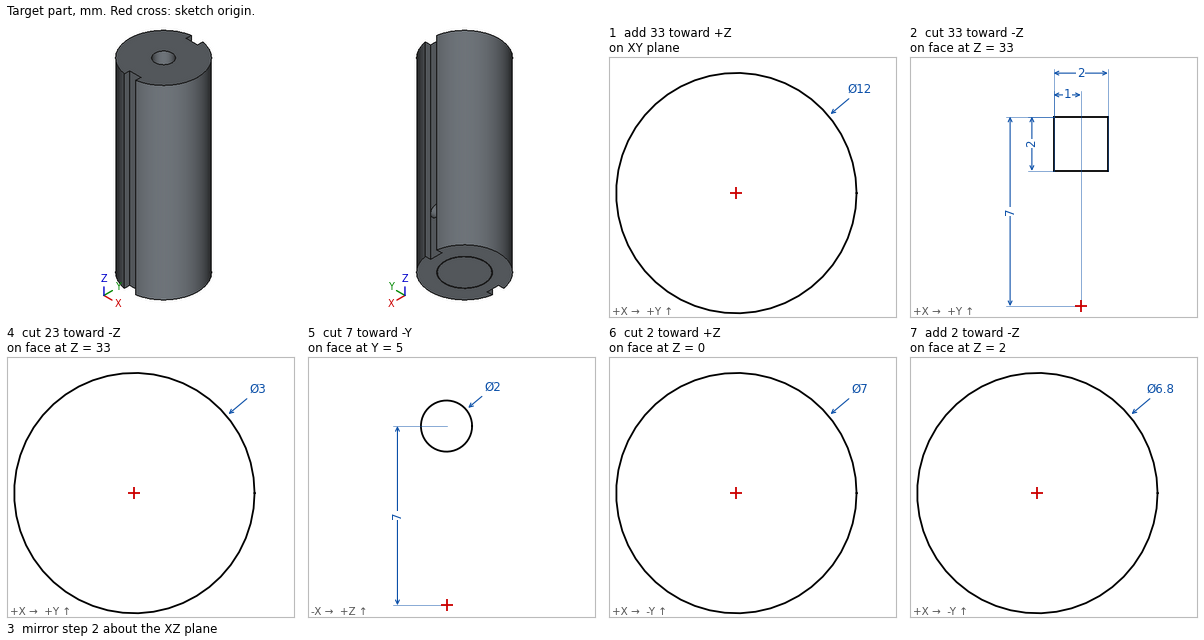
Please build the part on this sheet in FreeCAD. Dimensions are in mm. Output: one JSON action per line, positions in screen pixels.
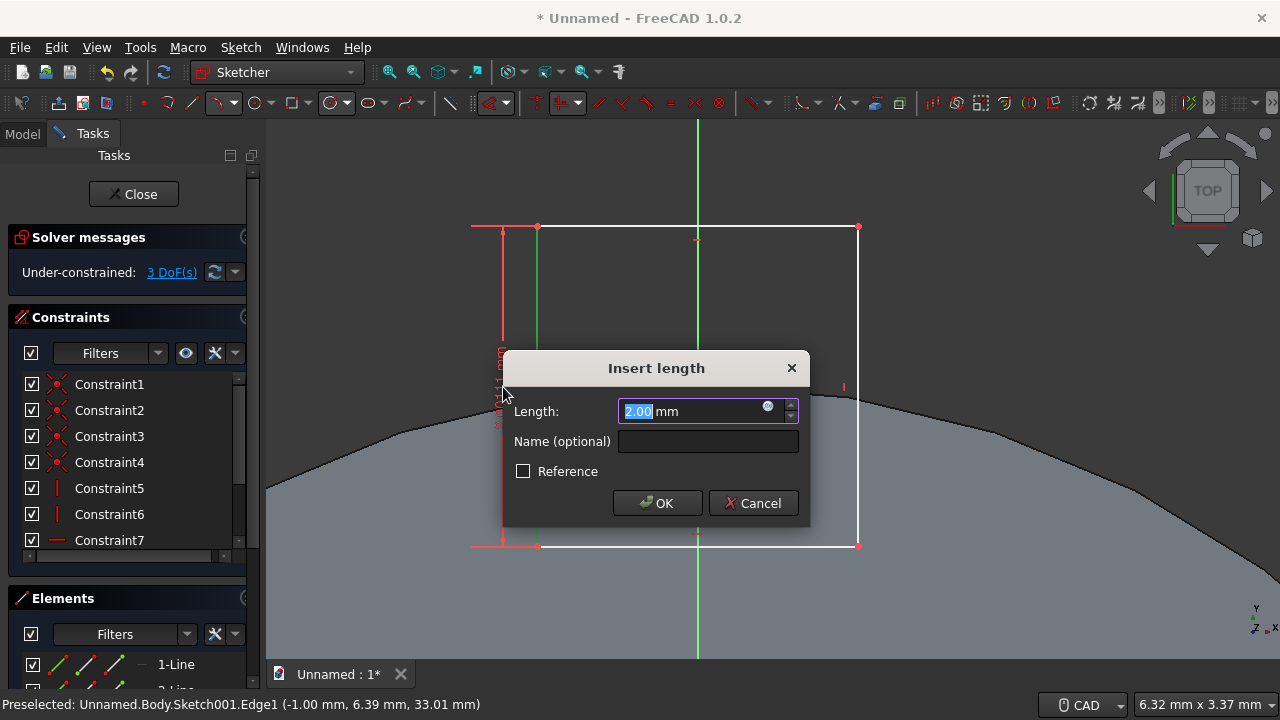
{"action": "type", "text": "2"}
{"action": "key", "text": "Return"}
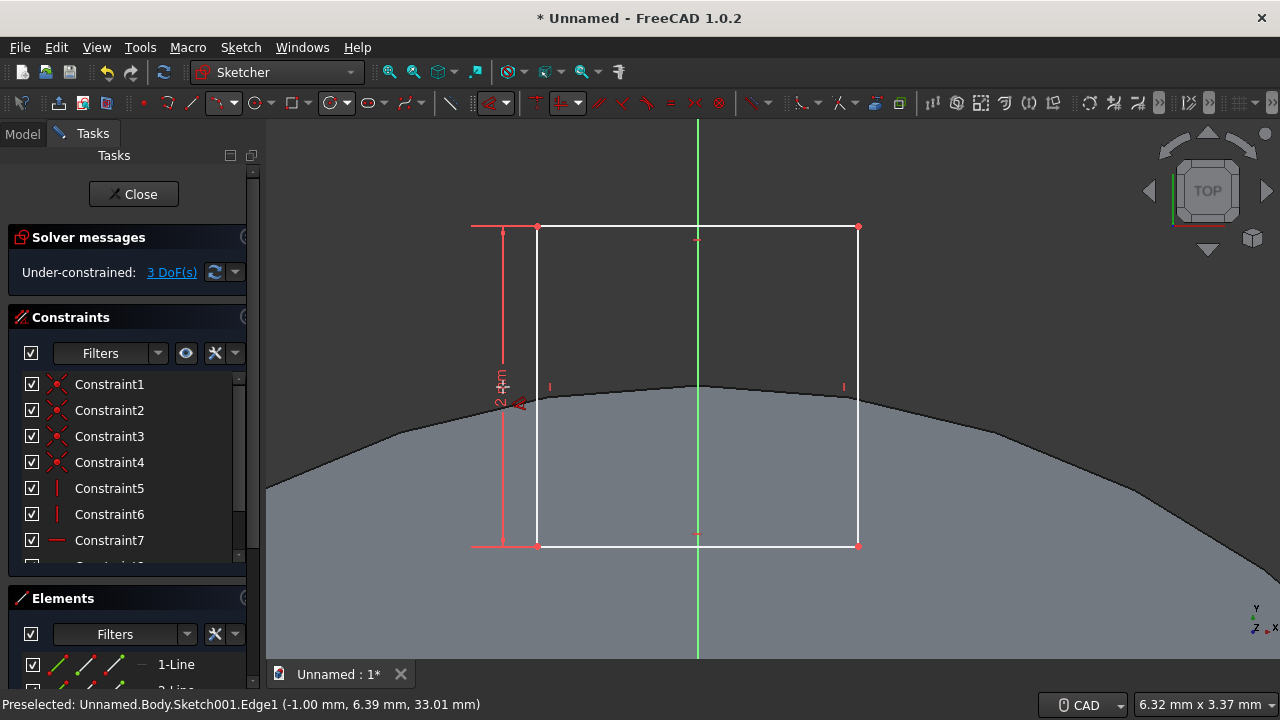
{"action": "left_click", "coordinate": [633, 547]}
{"action": "left_click", "coordinate": [624, 581]}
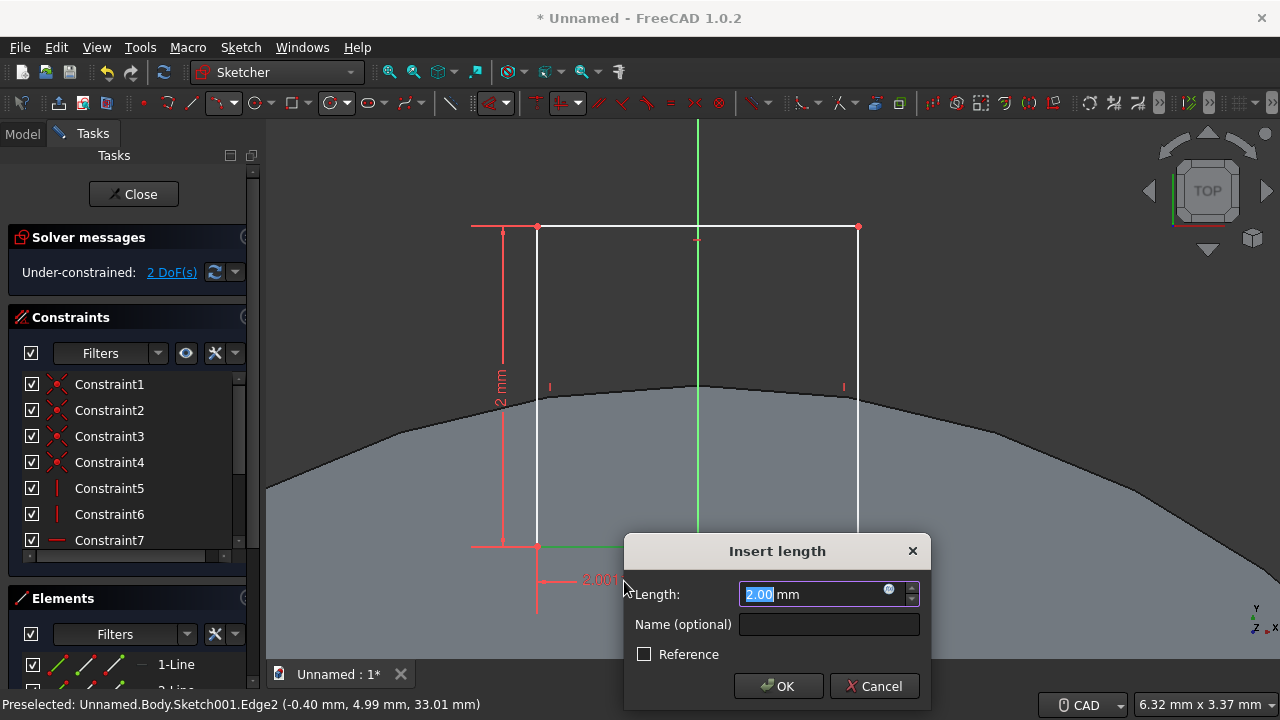
{"action": "type", "text": "2"}
{"action": "key", "text": "Return"}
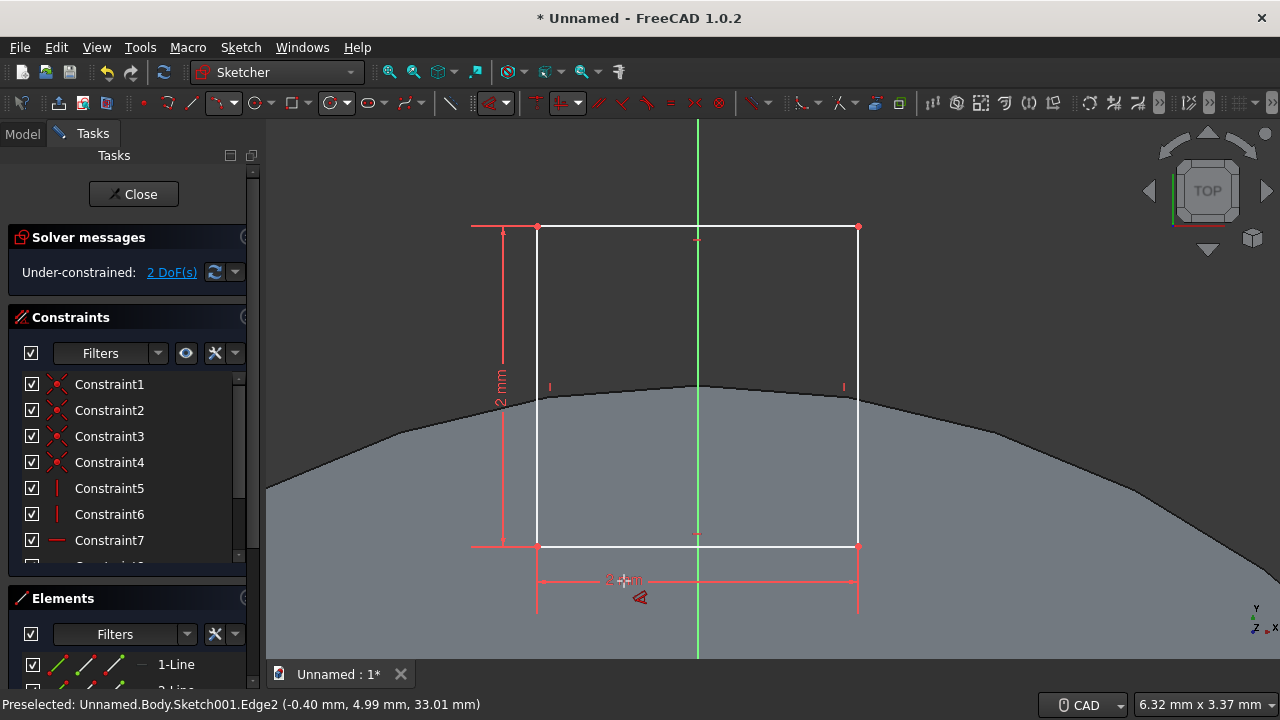
{"action": "left_click", "coordinate": [537, 226]}
{"action": "left_click", "coordinate": [617, 192]}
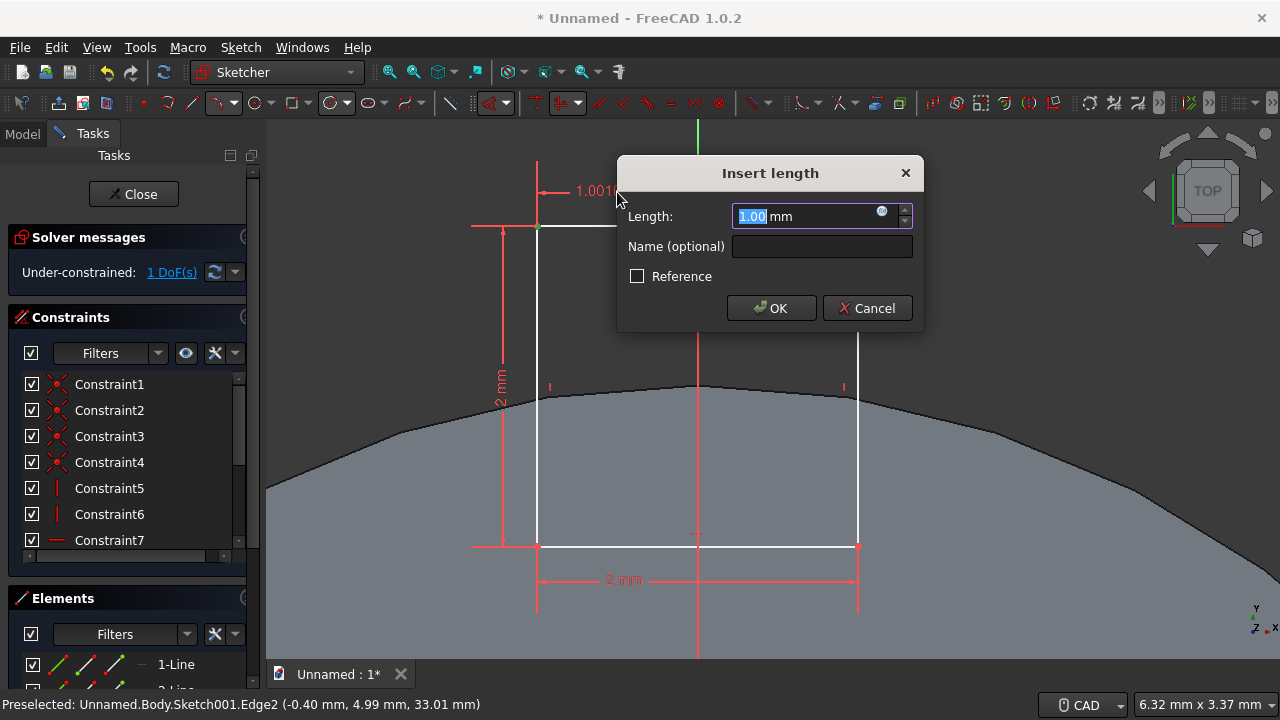
{"action": "type", "text": "1"}
{"action": "key", "text": "Return"}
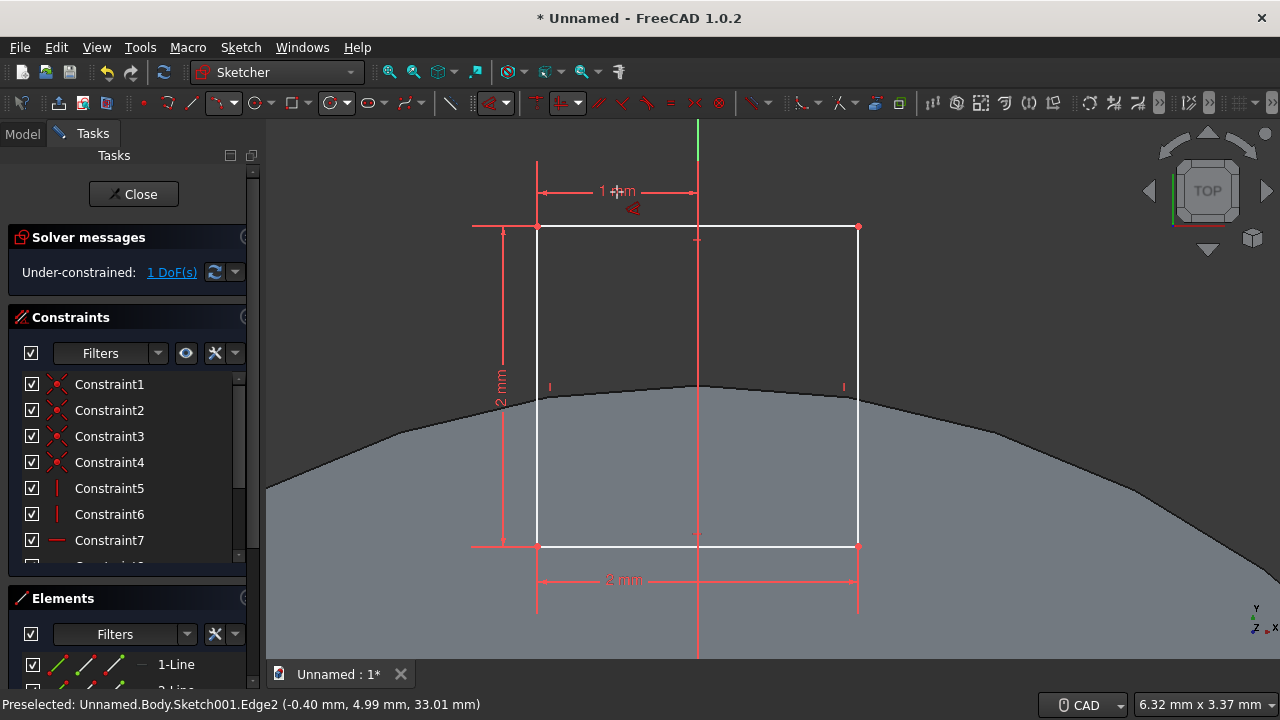
{"action": "left_click", "coordinate": [537, 226]}
{"action": "left_click", "coordinate": [503, 429]}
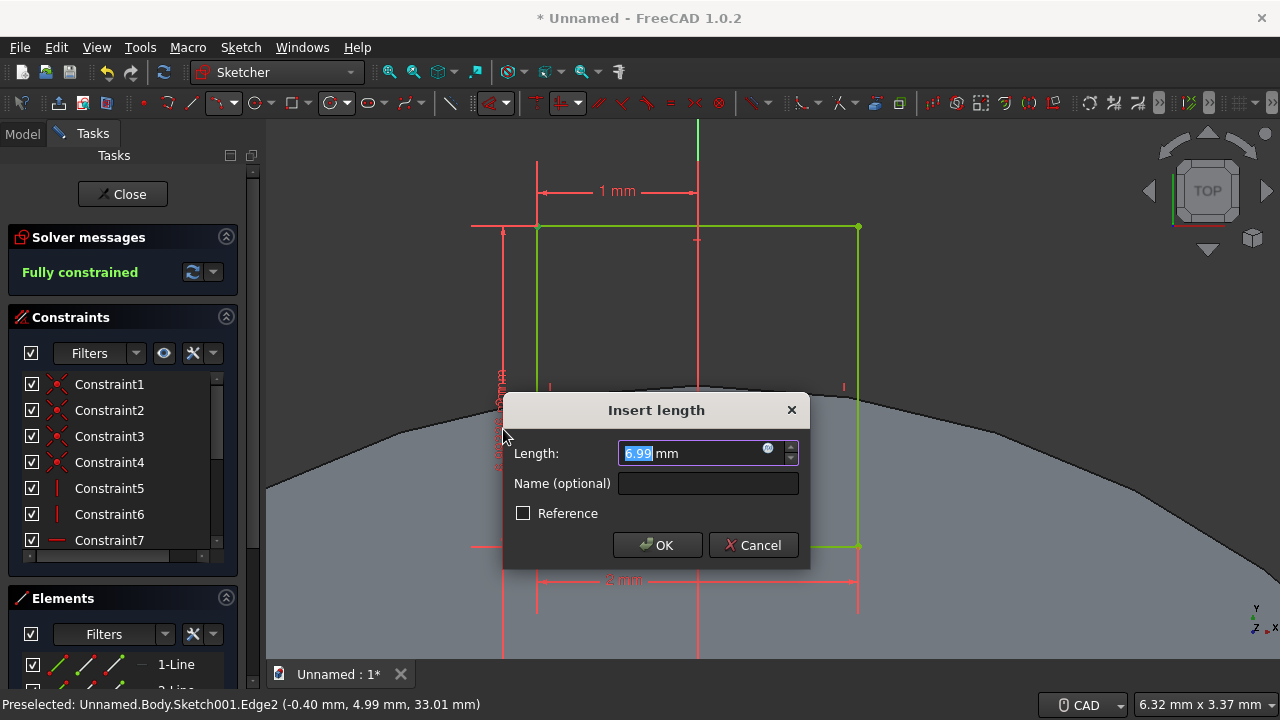
{"action": "type", "text": "7"}
{"action": "key", "text": "Return"}
{"action": "key", "text": "Escape"}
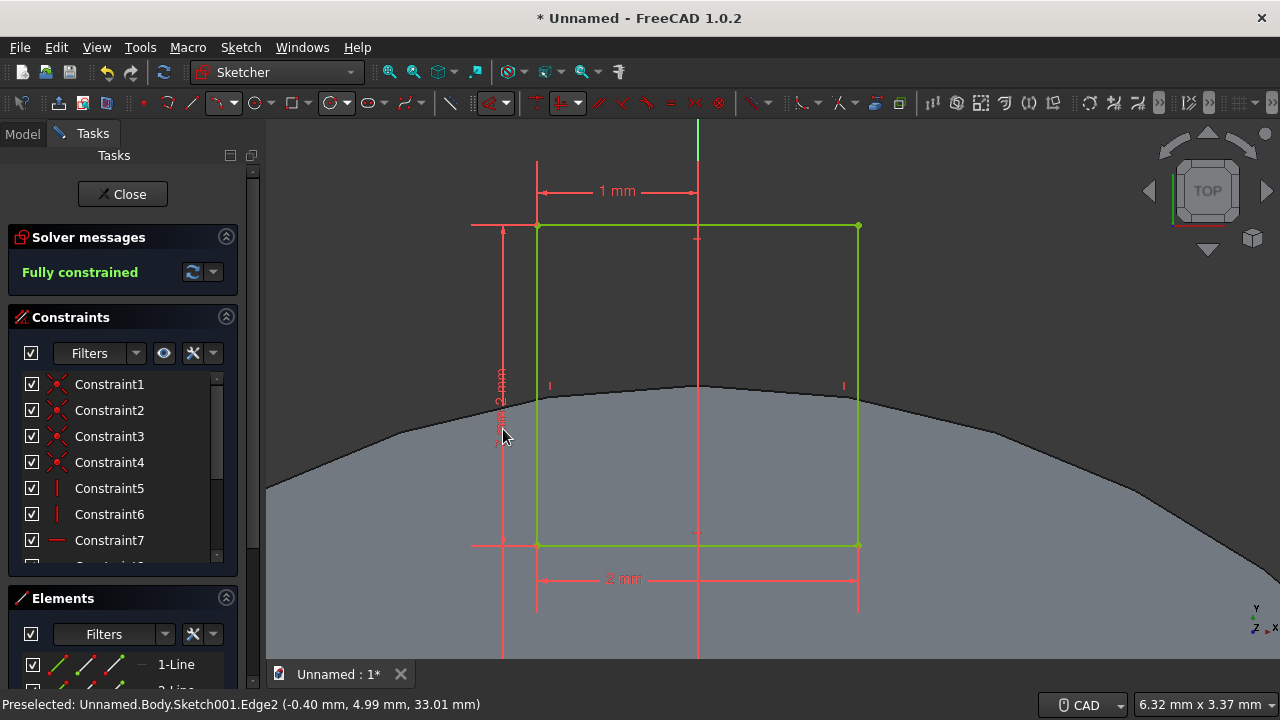
{"action": "left_click", "coordinate": [123, 194]}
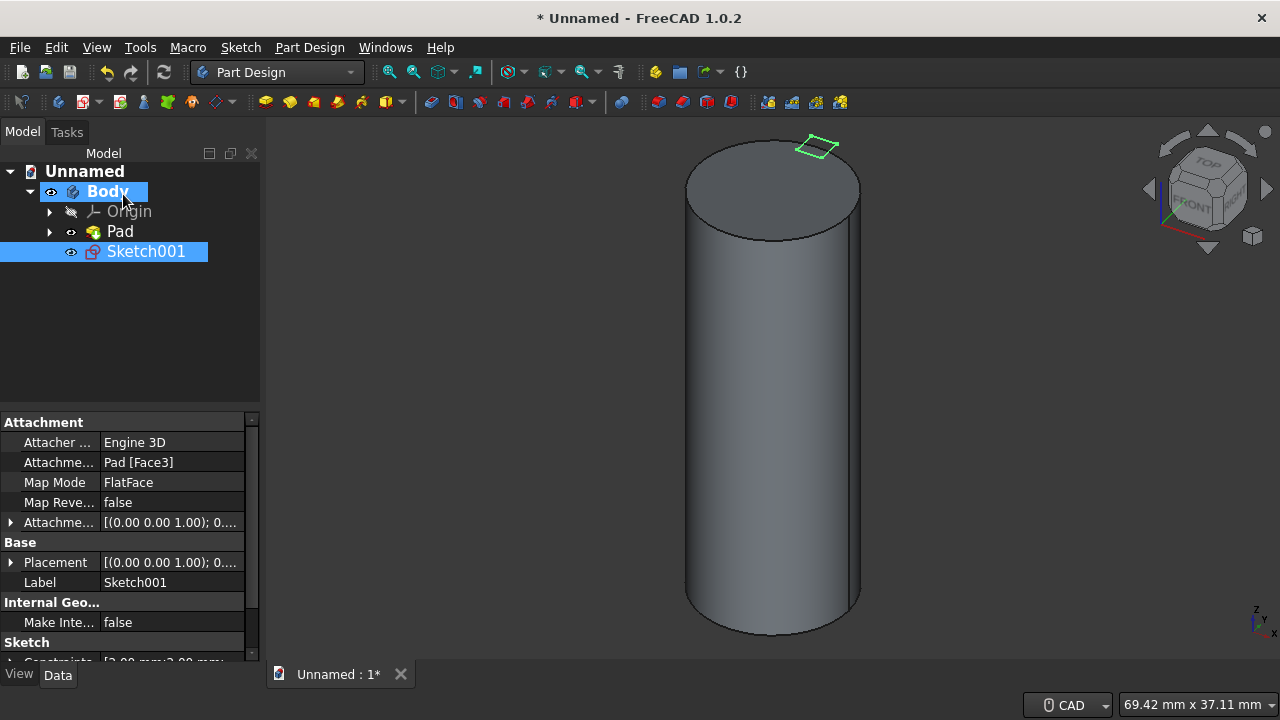
{"action": "left_click", "coordinate": [432, 102]}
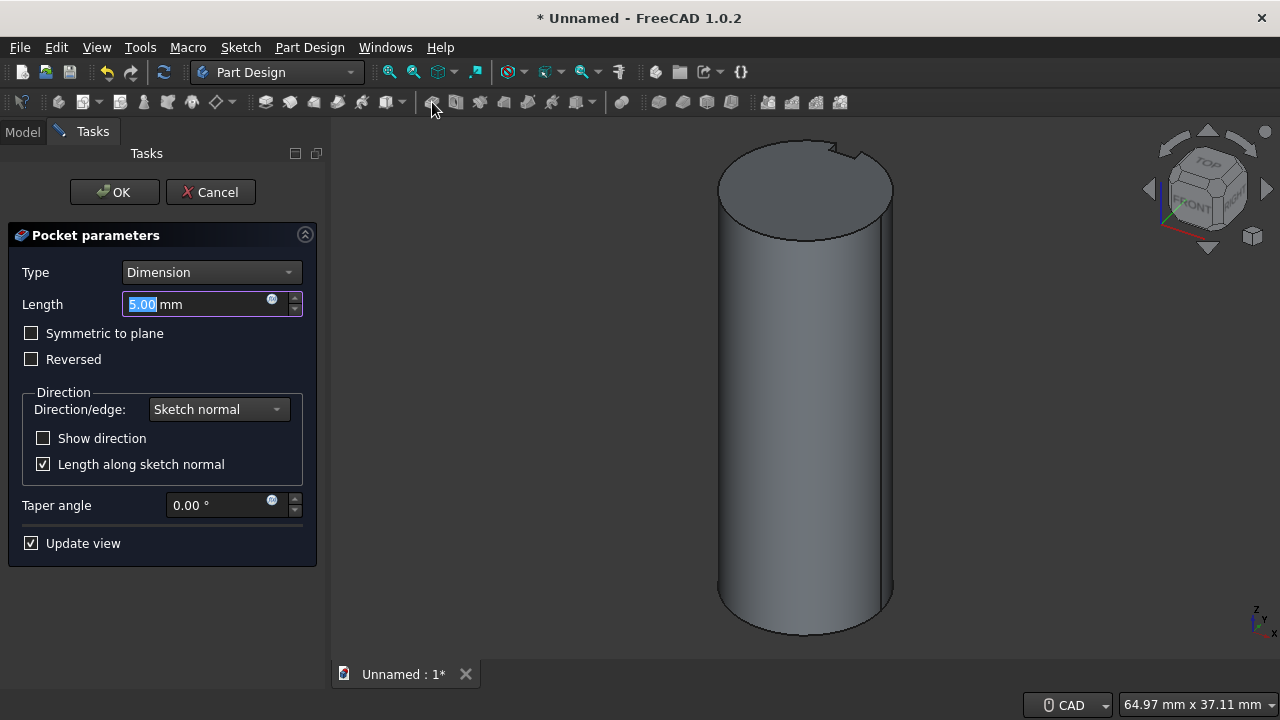
{"action": "type", "text": "33"}
{"action": "key", "text": "Tab"}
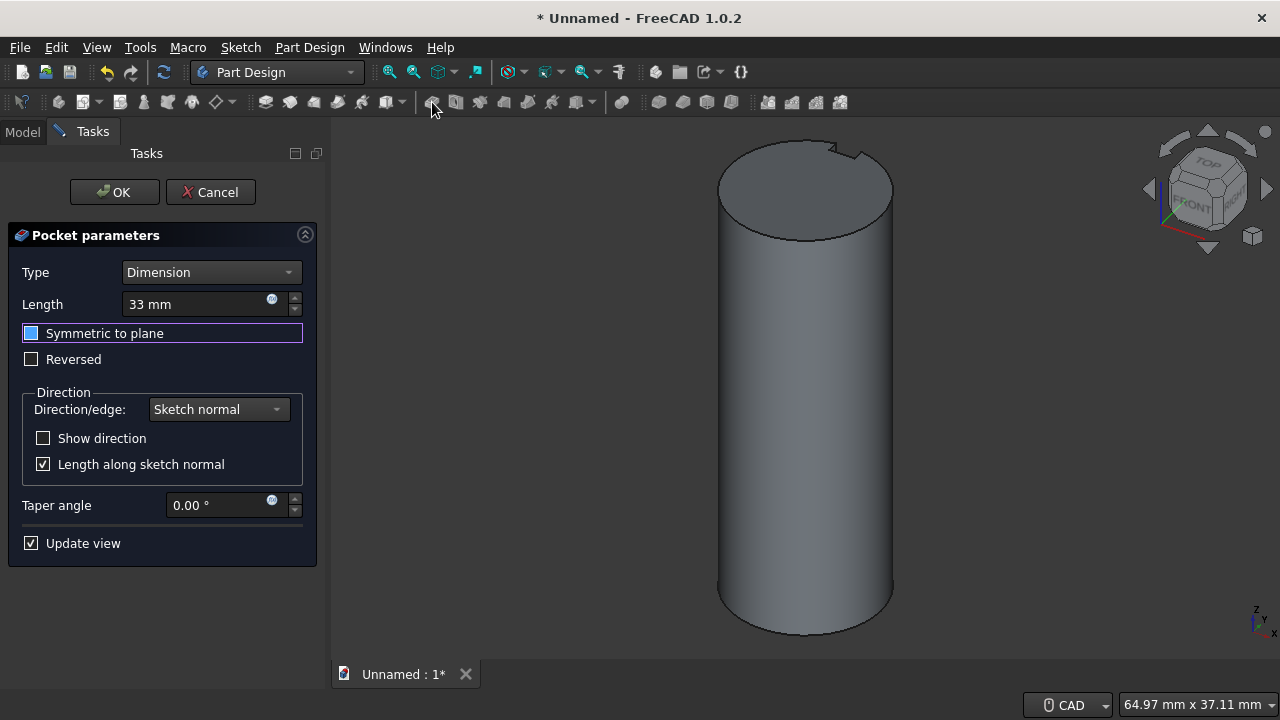
{"action": "left_click", "coordinate": [115, 192]}